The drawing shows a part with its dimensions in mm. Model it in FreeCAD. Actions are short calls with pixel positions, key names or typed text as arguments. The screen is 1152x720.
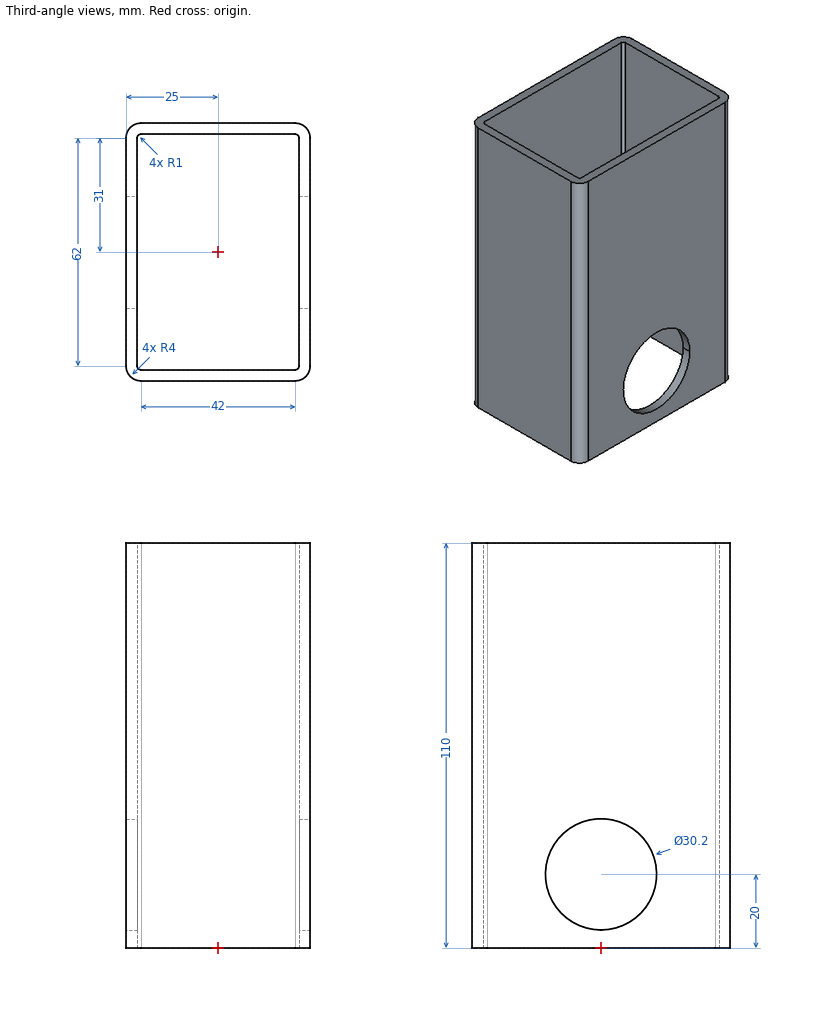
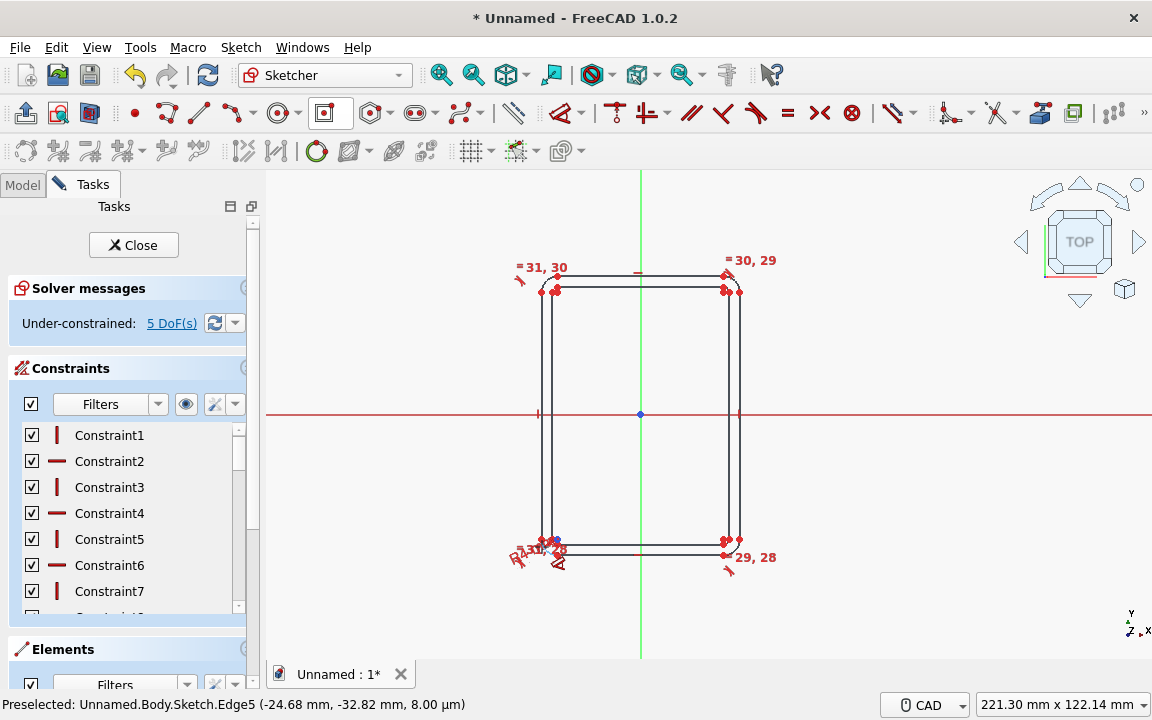
scroll(554, 289, up, 12)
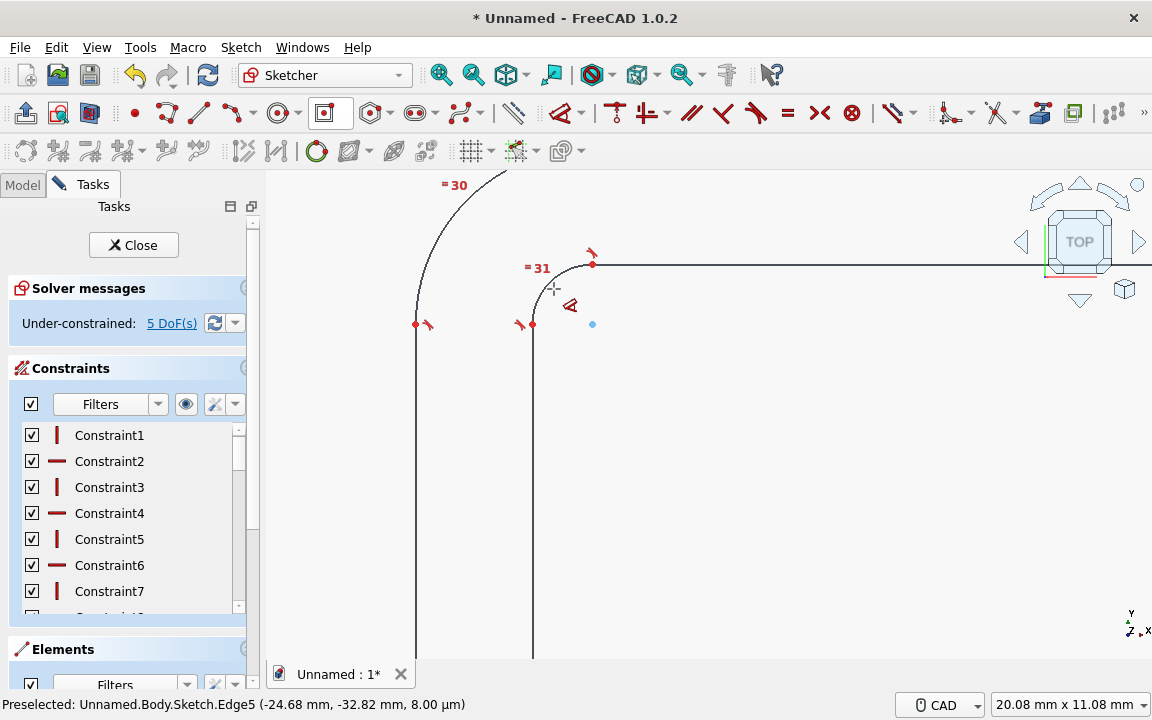
click(550, 282)
click(527, 259)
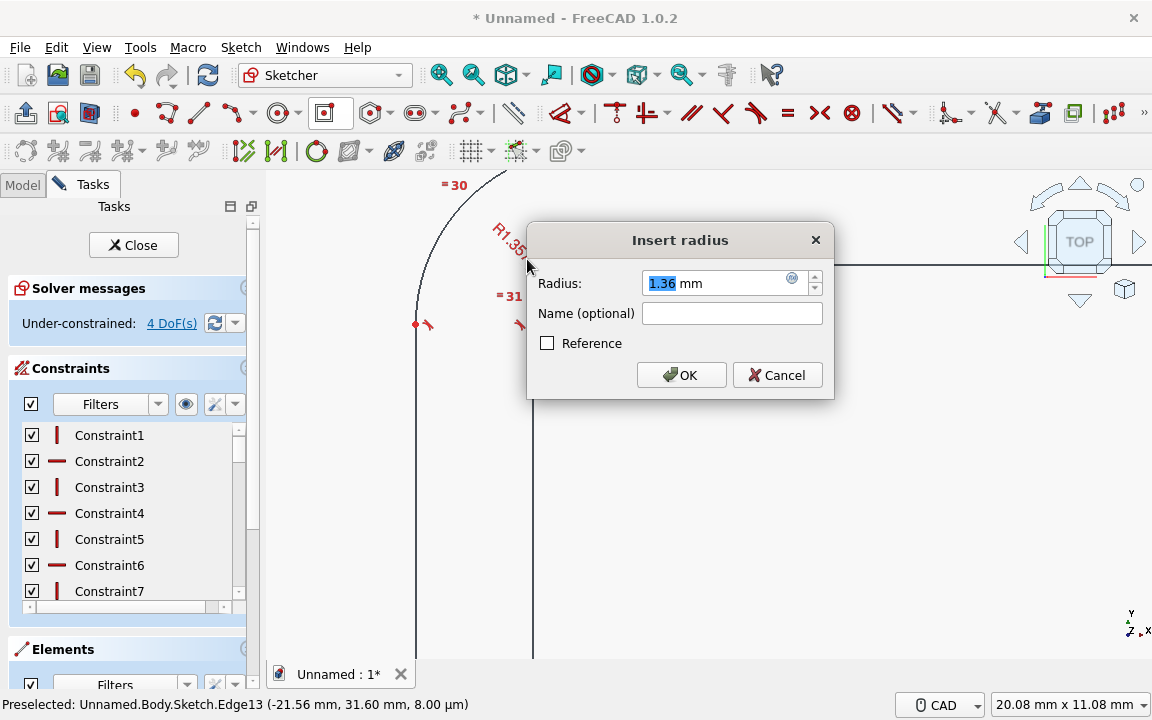
text(1)
key(Return)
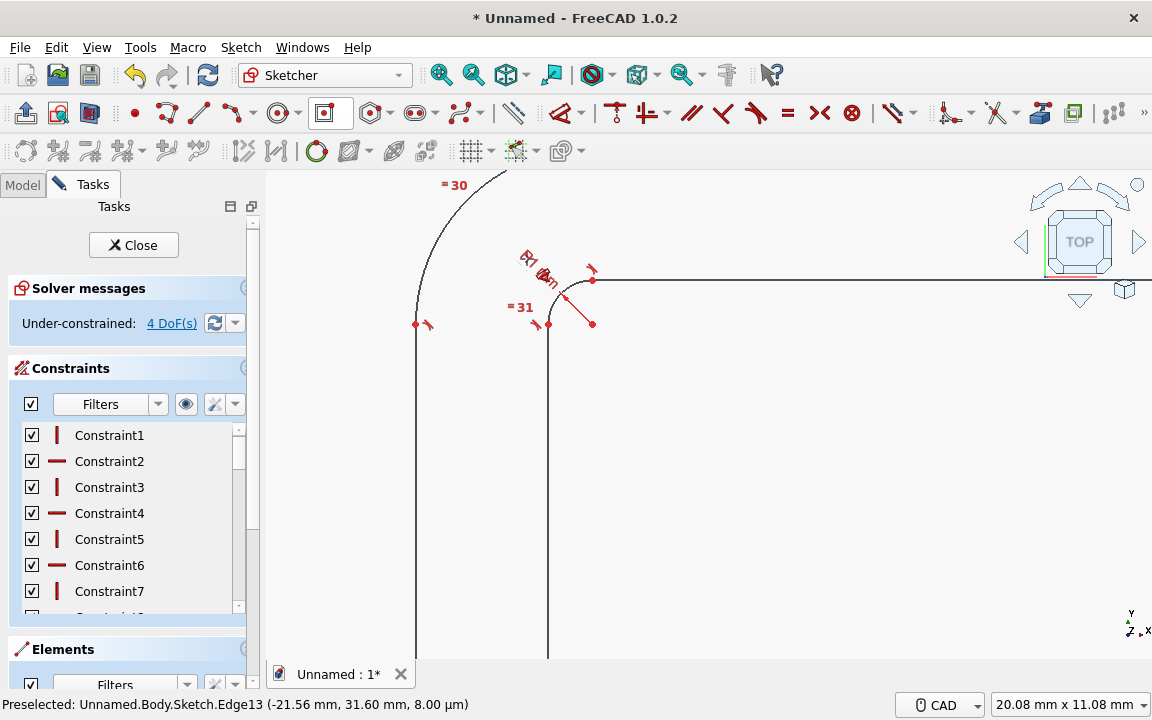
scroll(554, 289, down, 12)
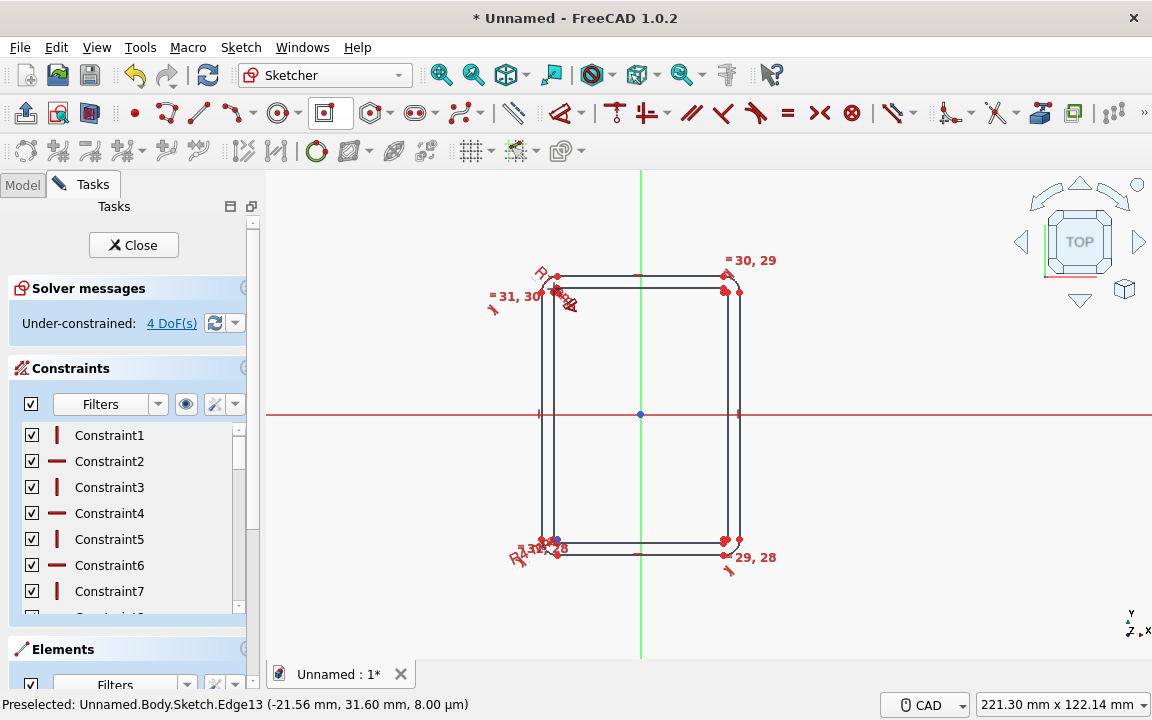
click(542, 367)
click(508, 359)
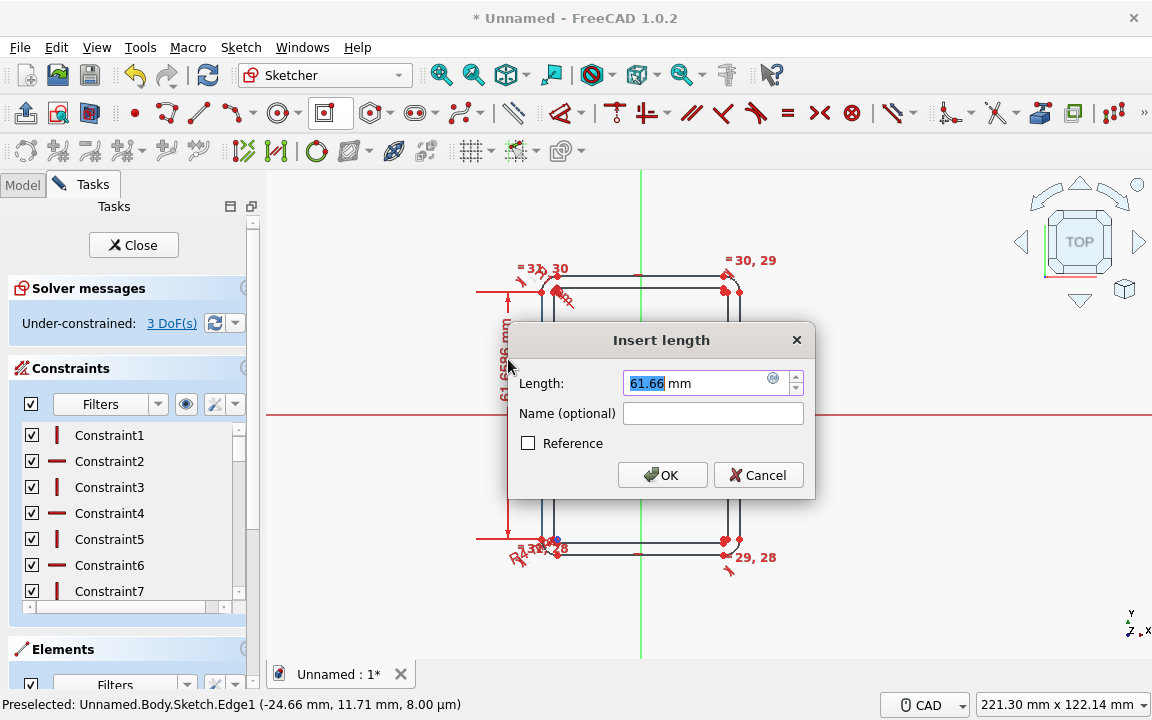
text(62)
key(Return)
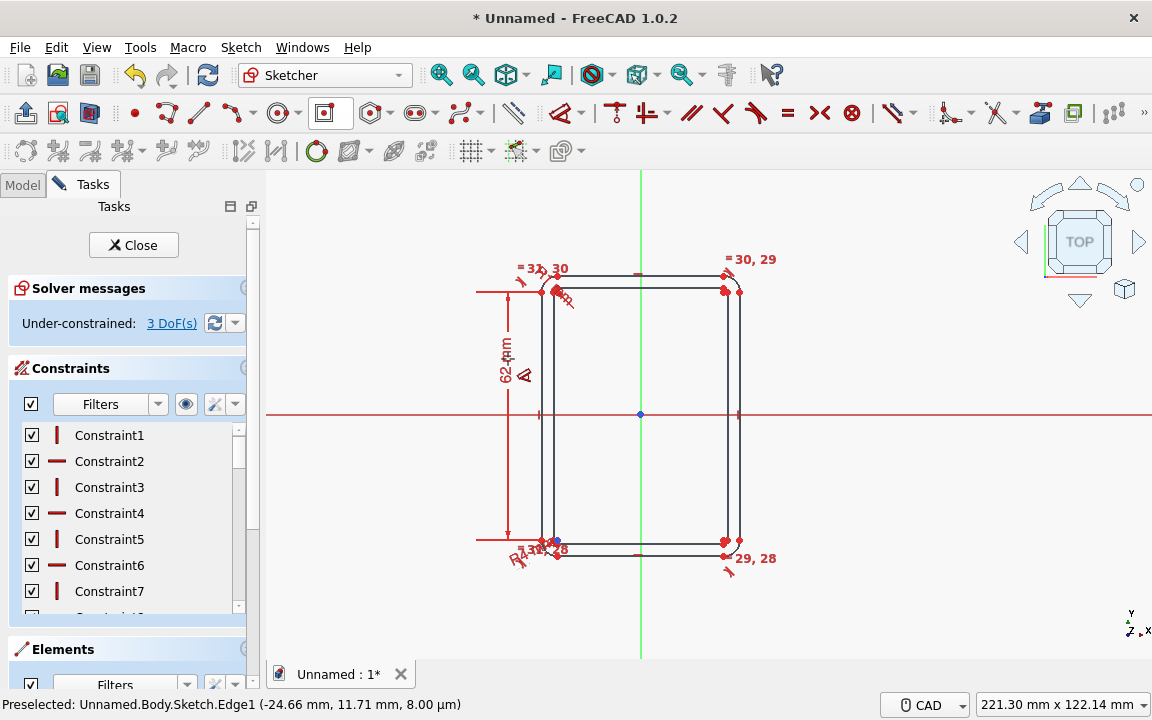
click(608, 556)
click(603, 590)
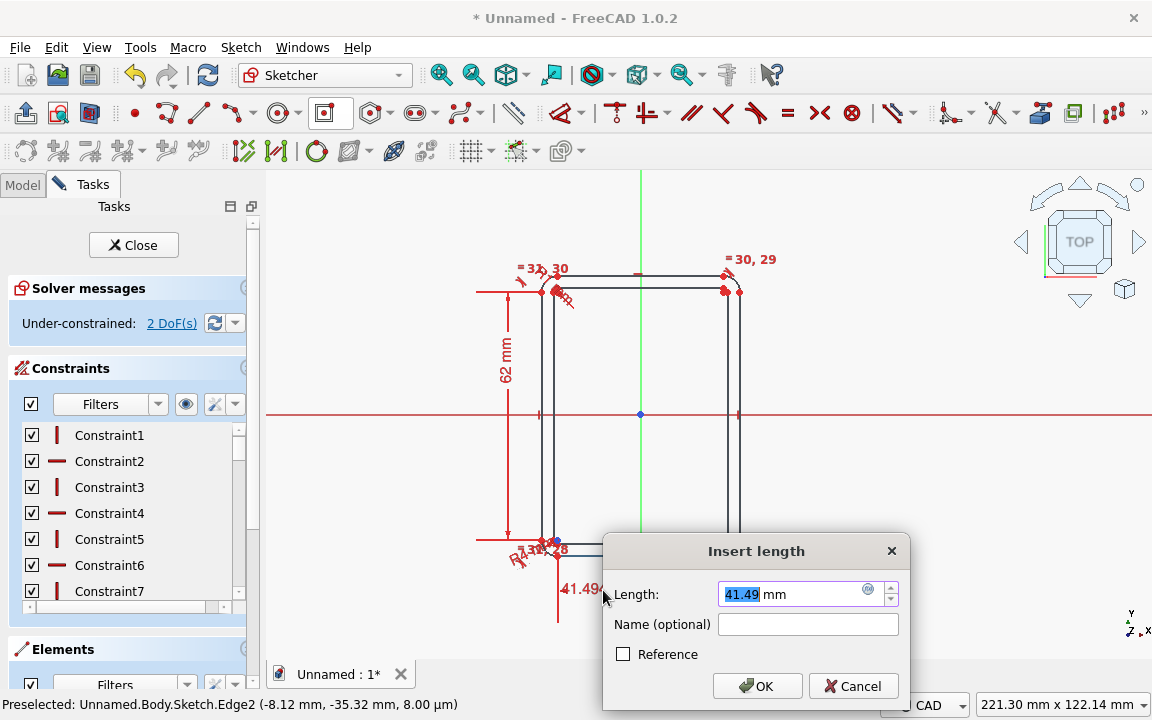
text(42)
key(Return)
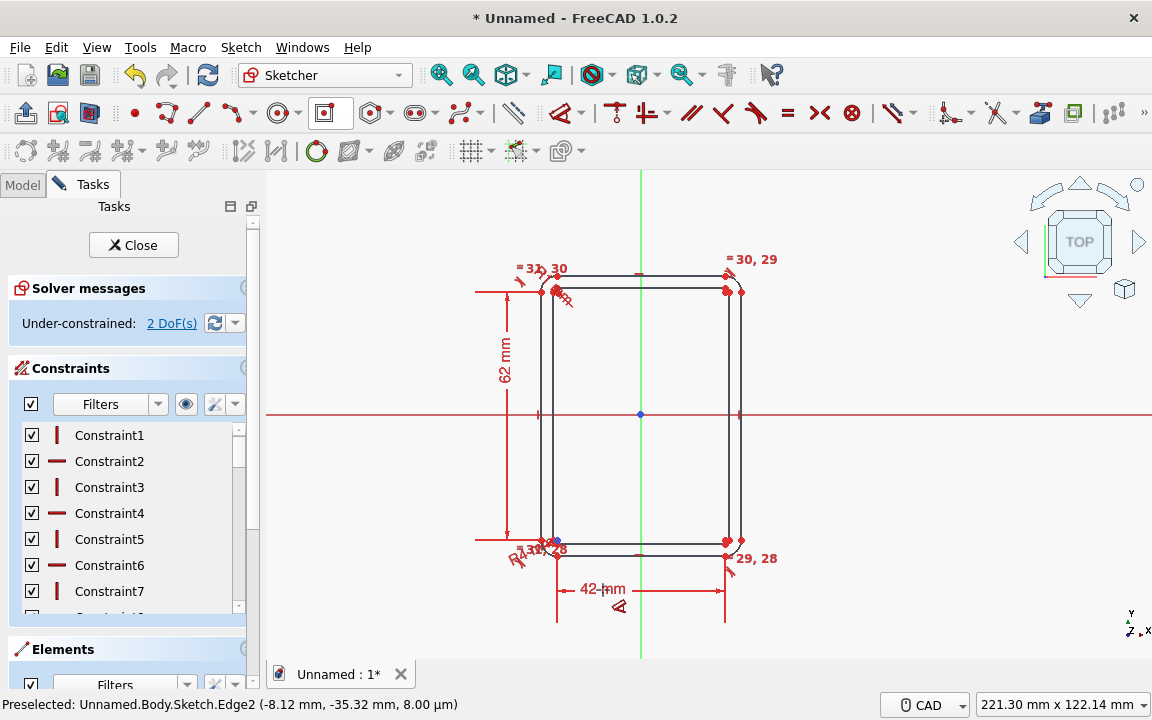
click(541, 292)
click(591, 258)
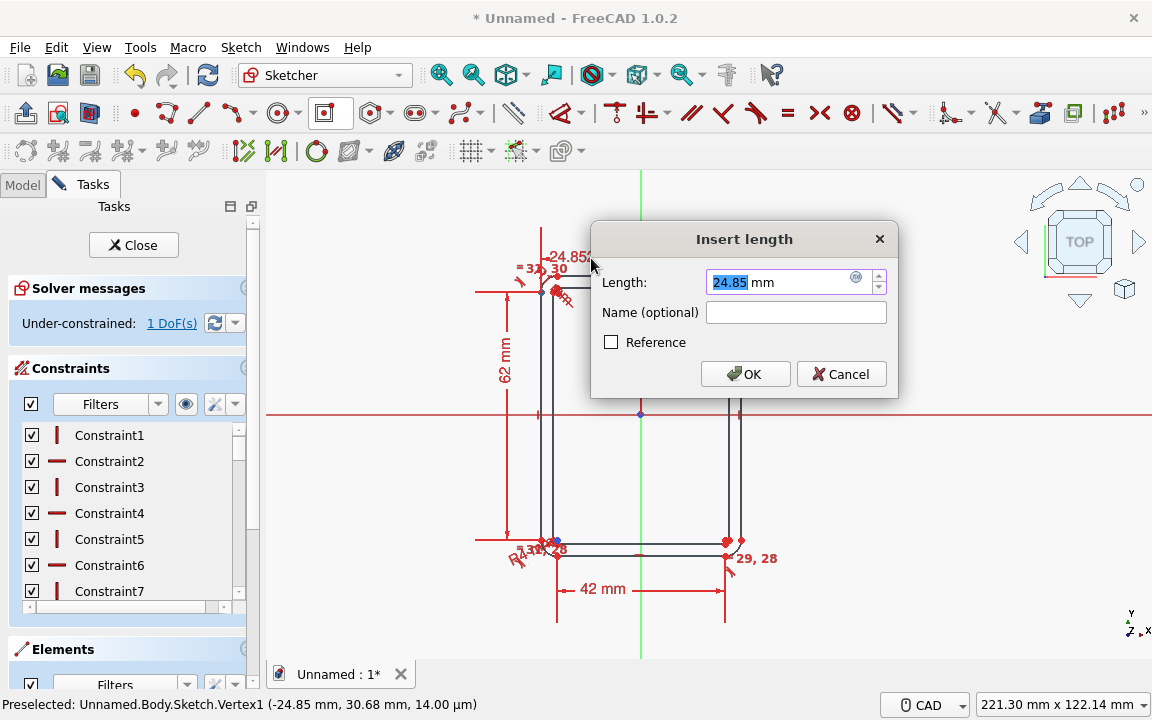
text(25)
key(Return)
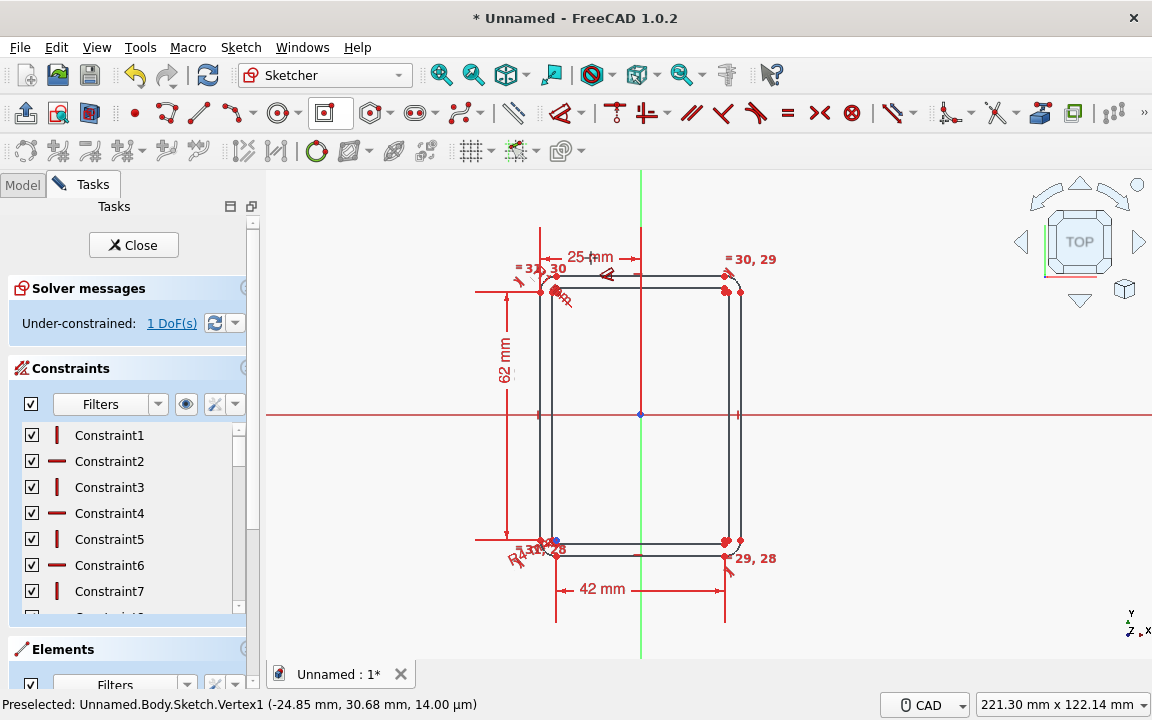
click(540, 292)
click(506, 325)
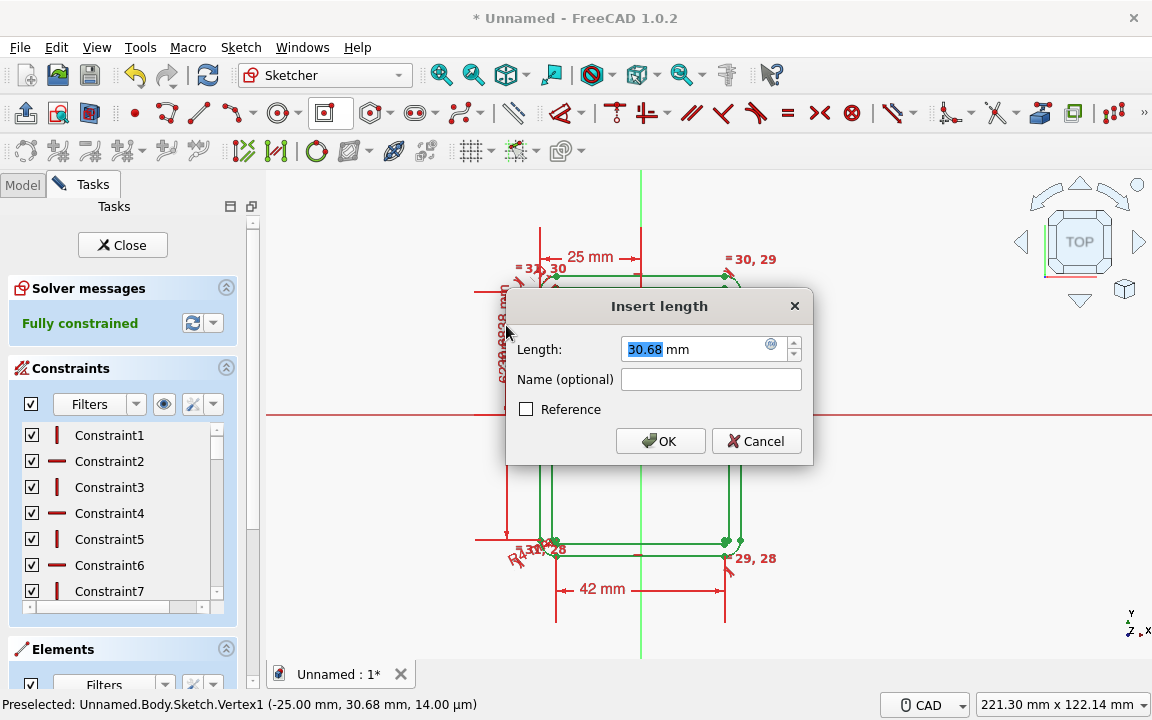
text(31)
key(Return)
key(Escape)